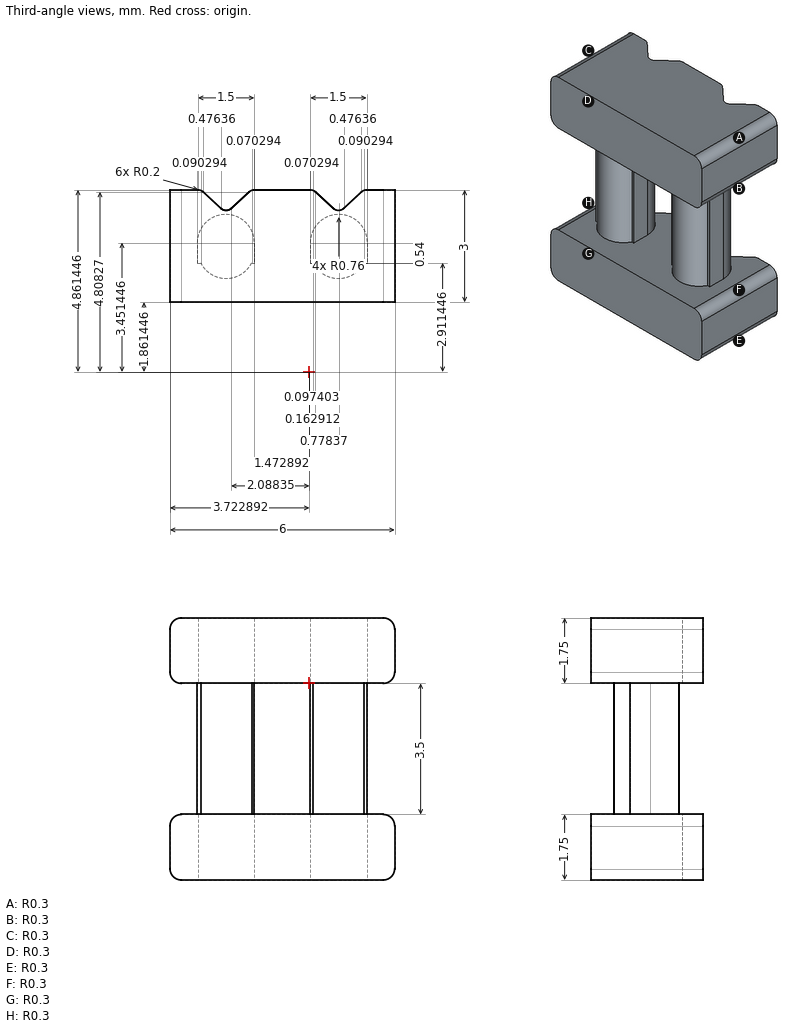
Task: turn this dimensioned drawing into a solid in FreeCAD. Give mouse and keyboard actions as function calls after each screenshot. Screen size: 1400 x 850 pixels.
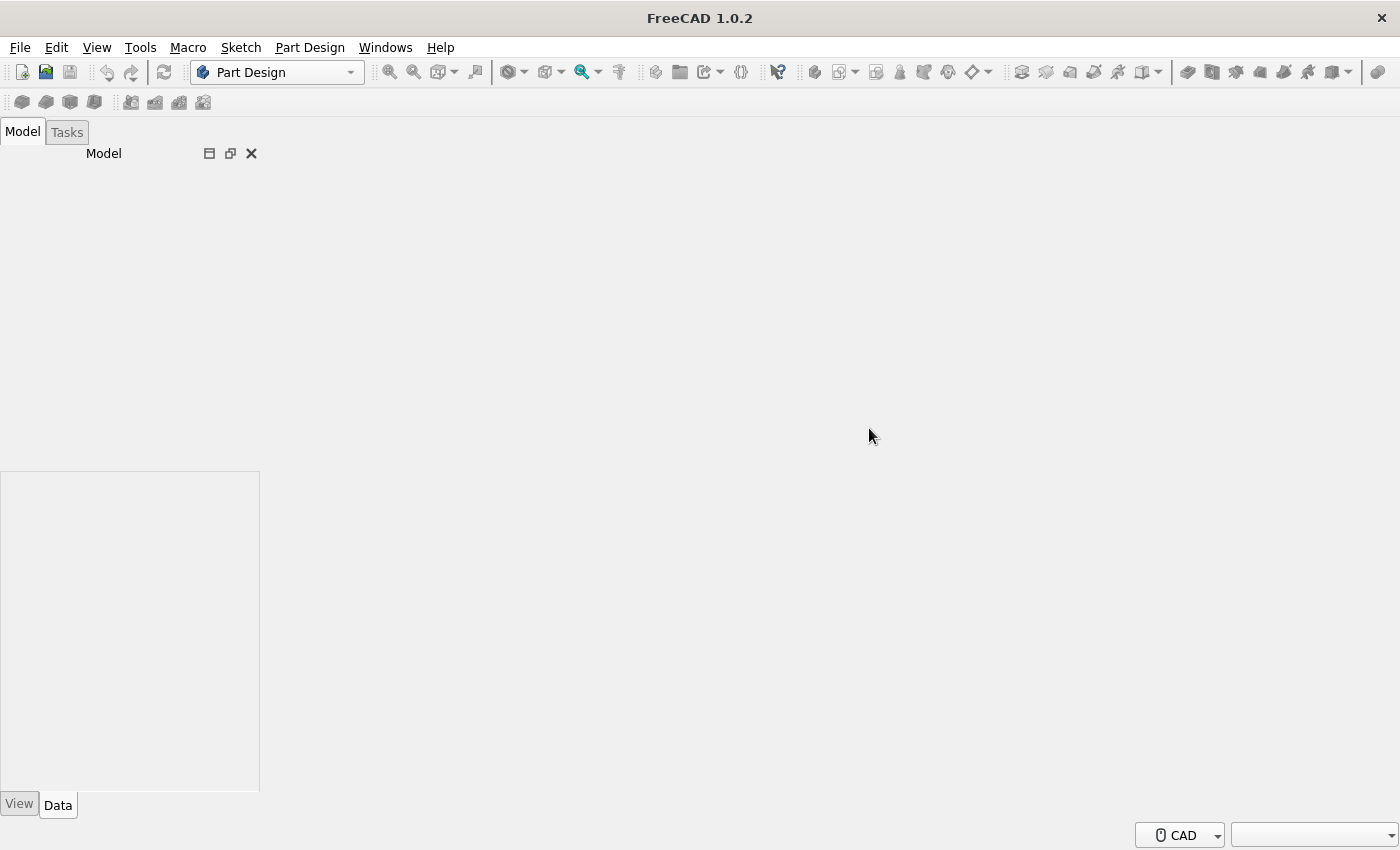
key(ctrl+n)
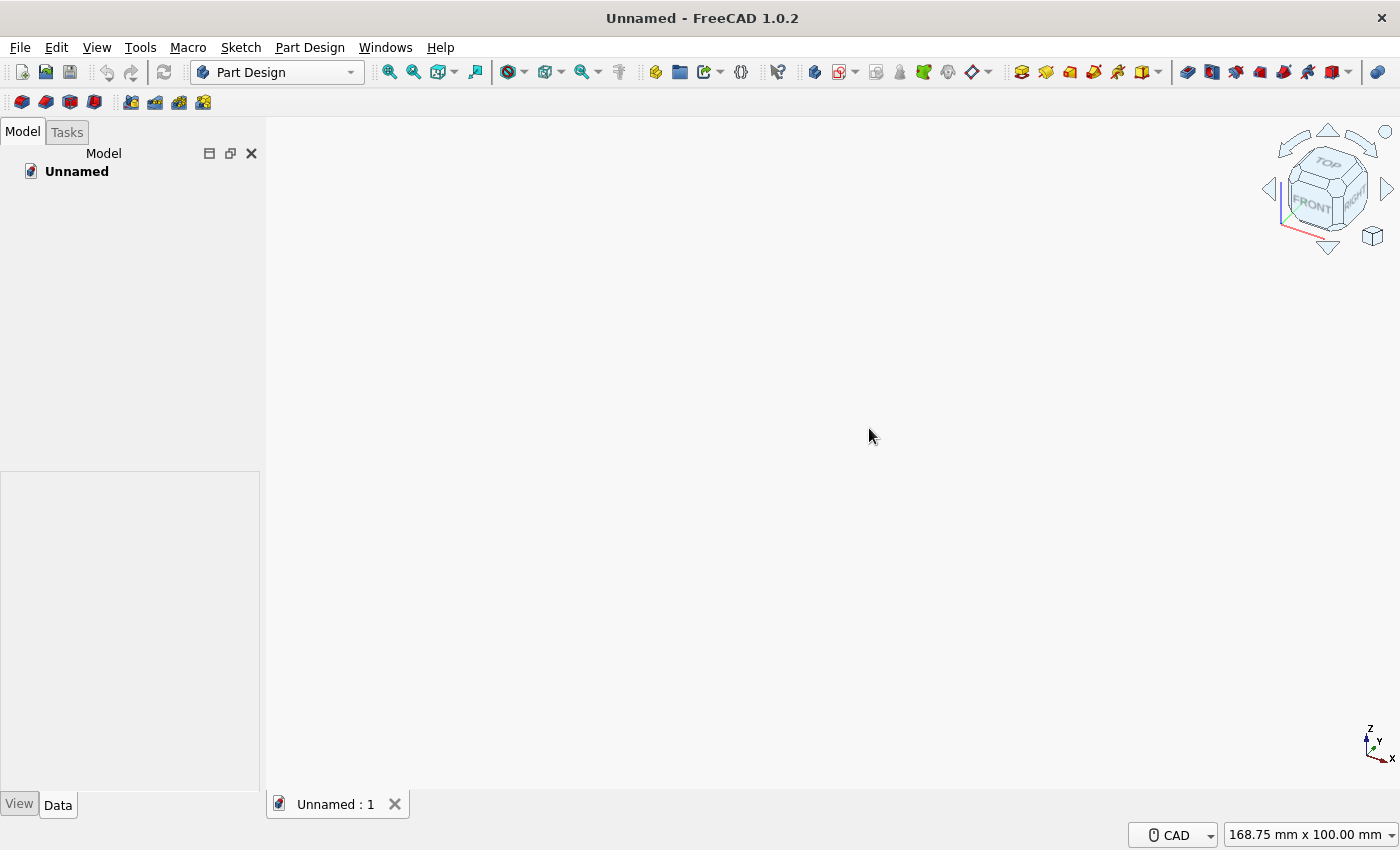
click(840, 72)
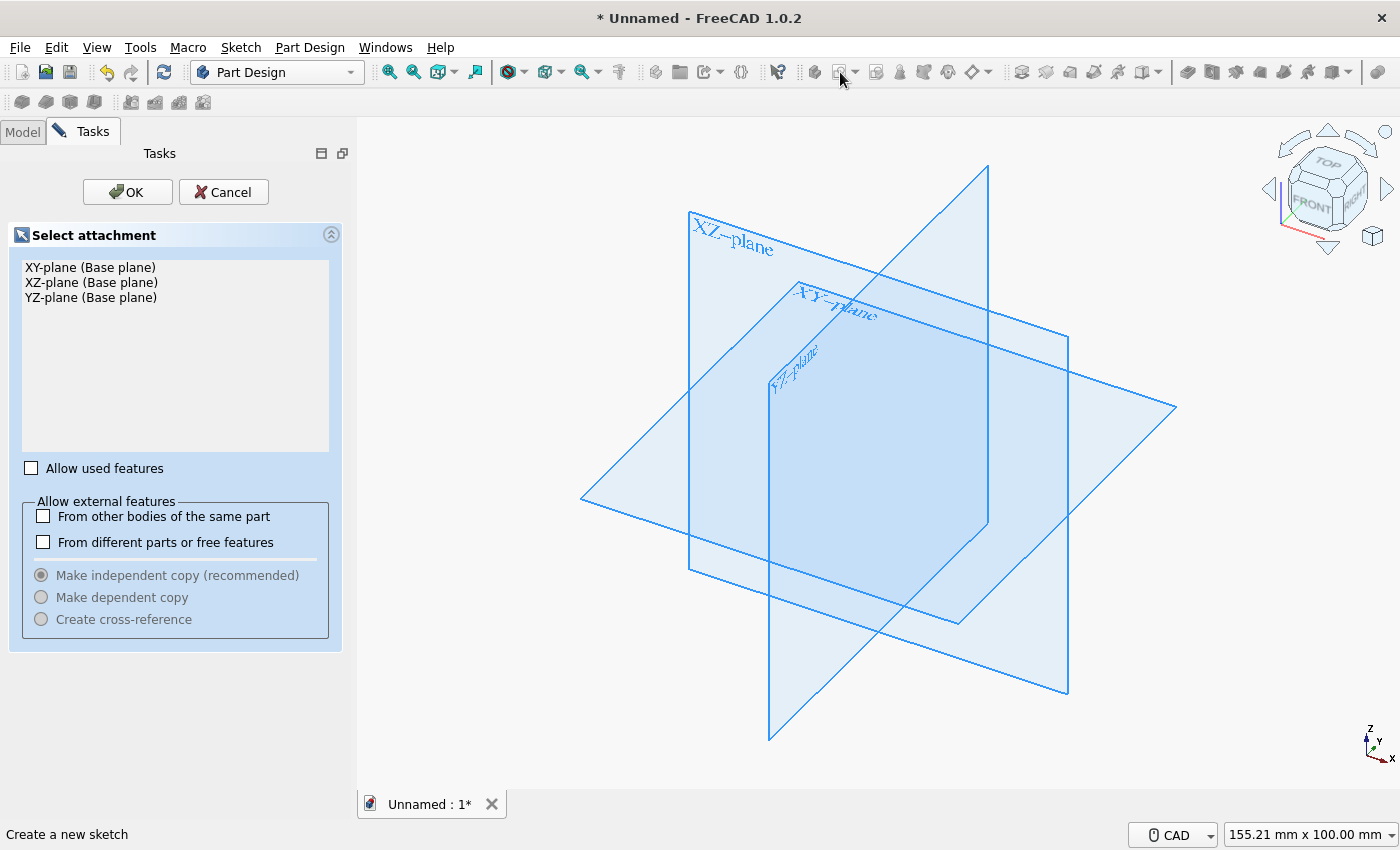
click(82, 268)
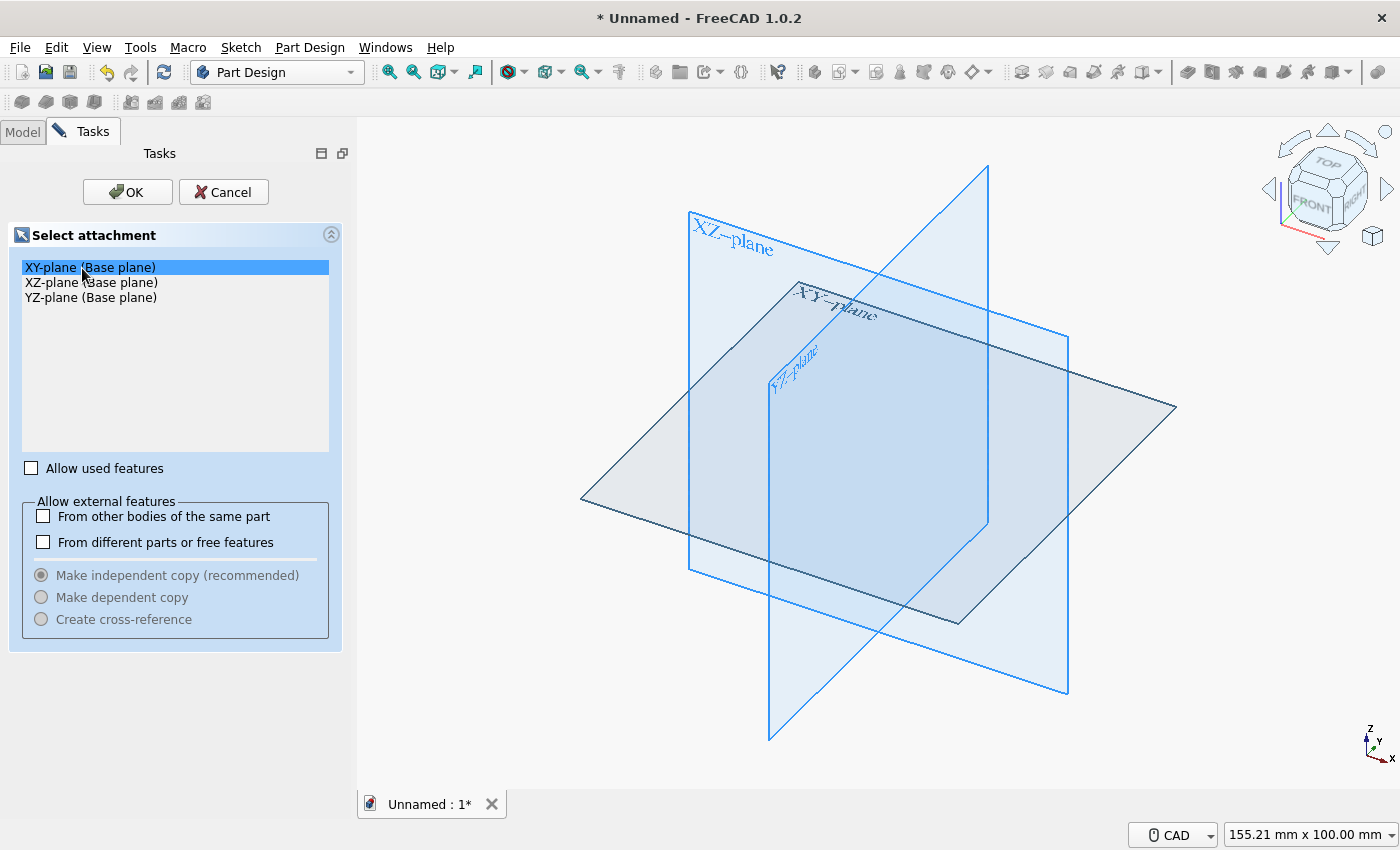
click(128, 192)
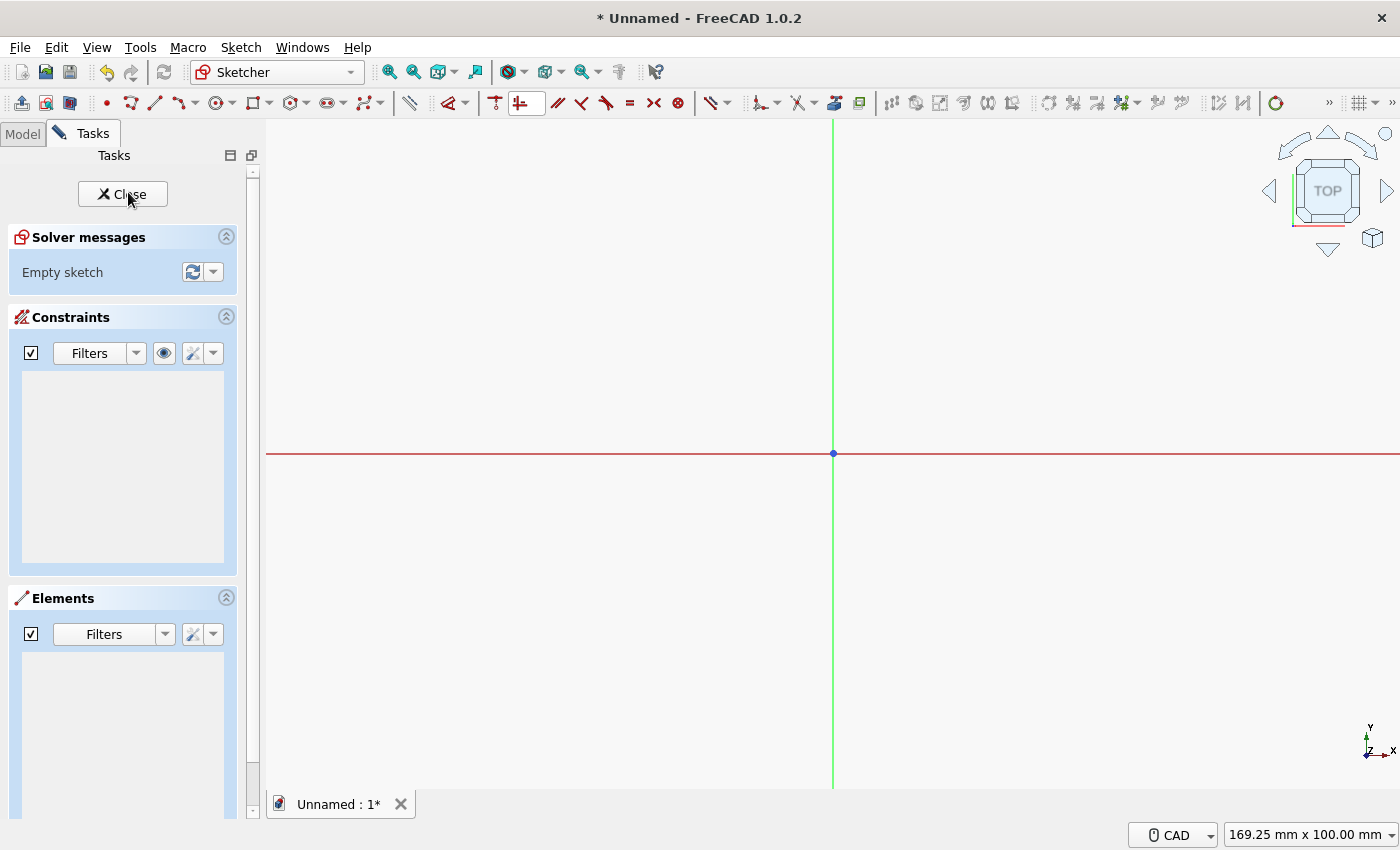
scroll(833, 436, up, 13)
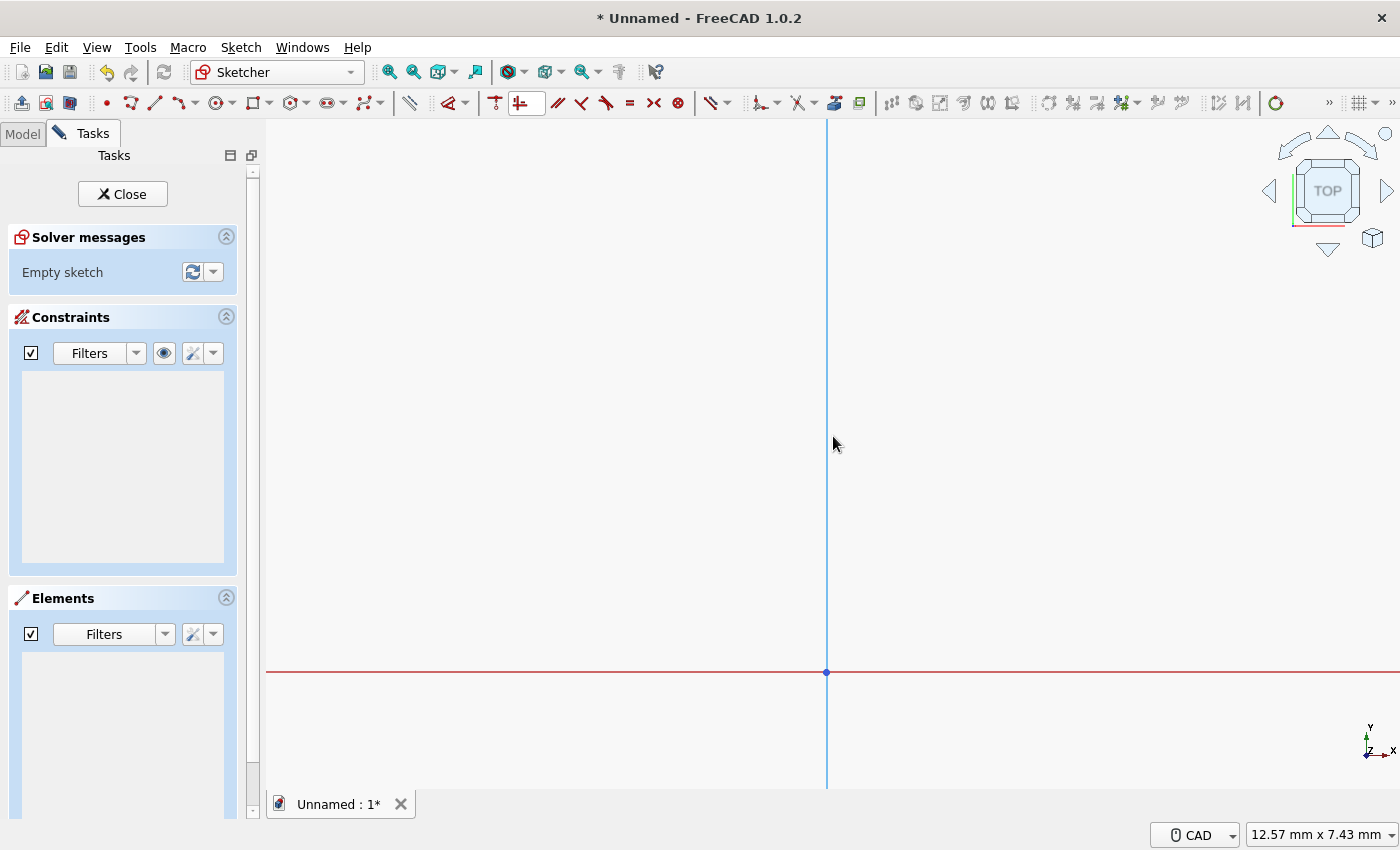
click(254, 104)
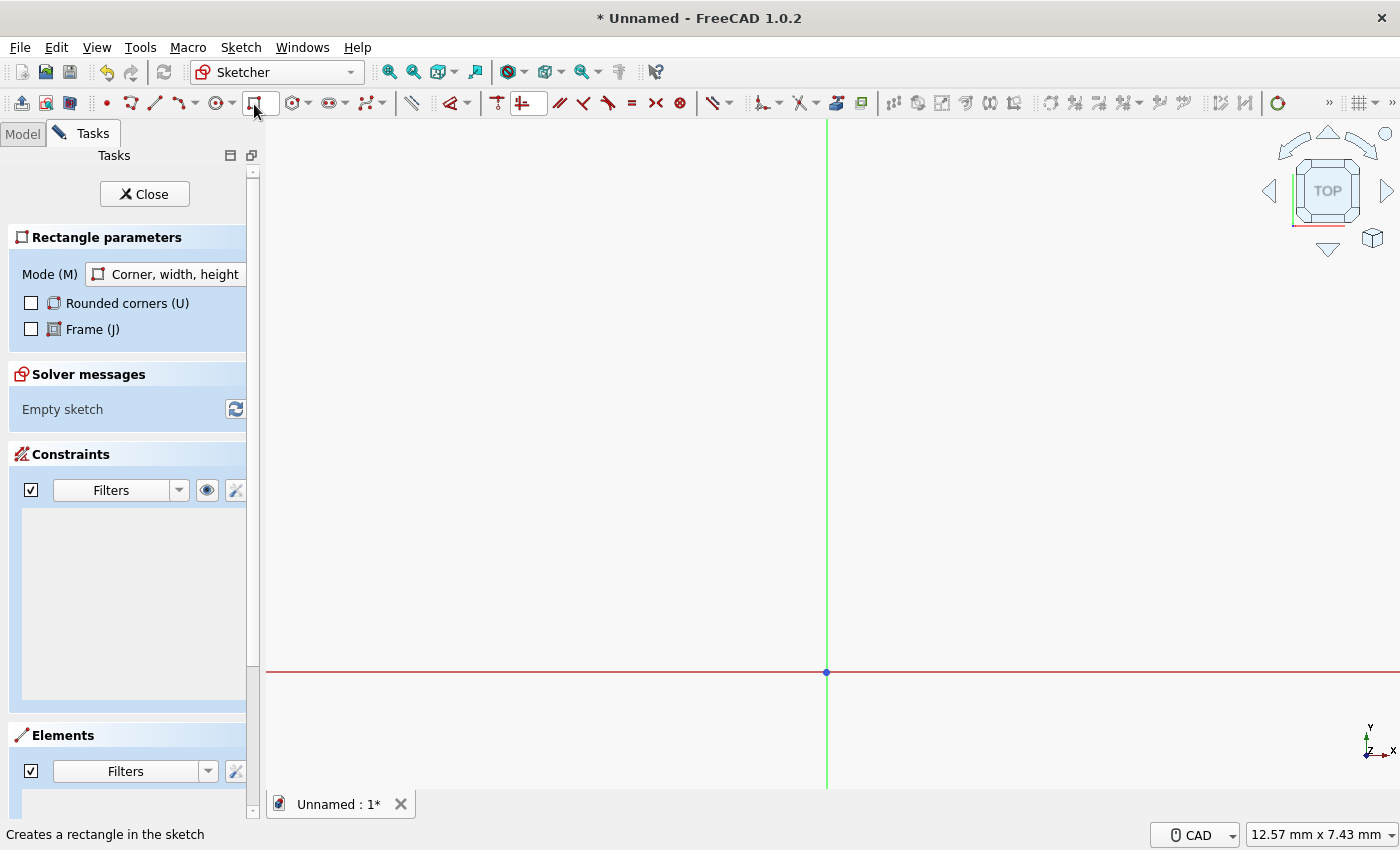
click(491, 234)
move(1032, 505)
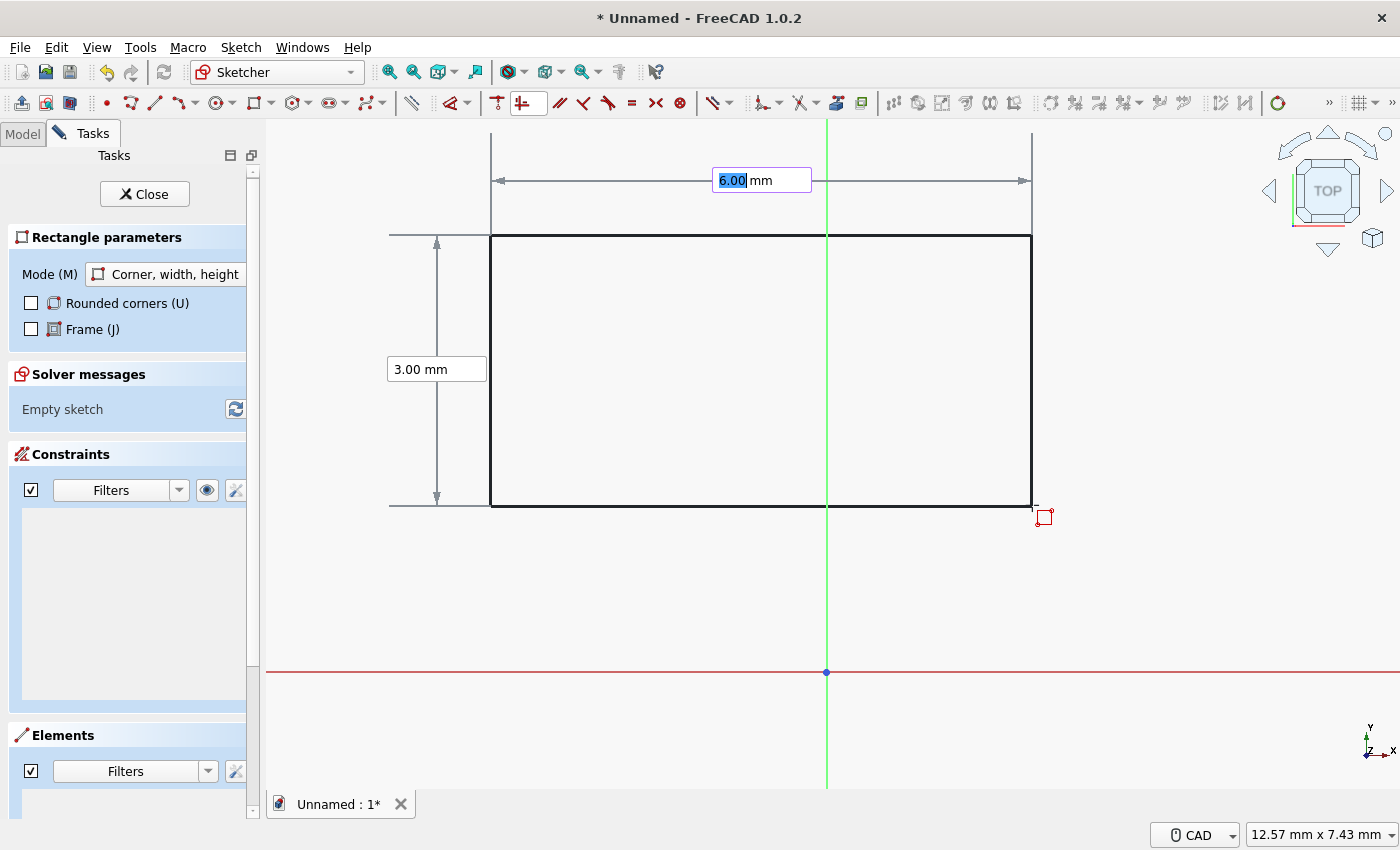
text(6)
key(Tab)
text(3)
key(Return)
key(Escape)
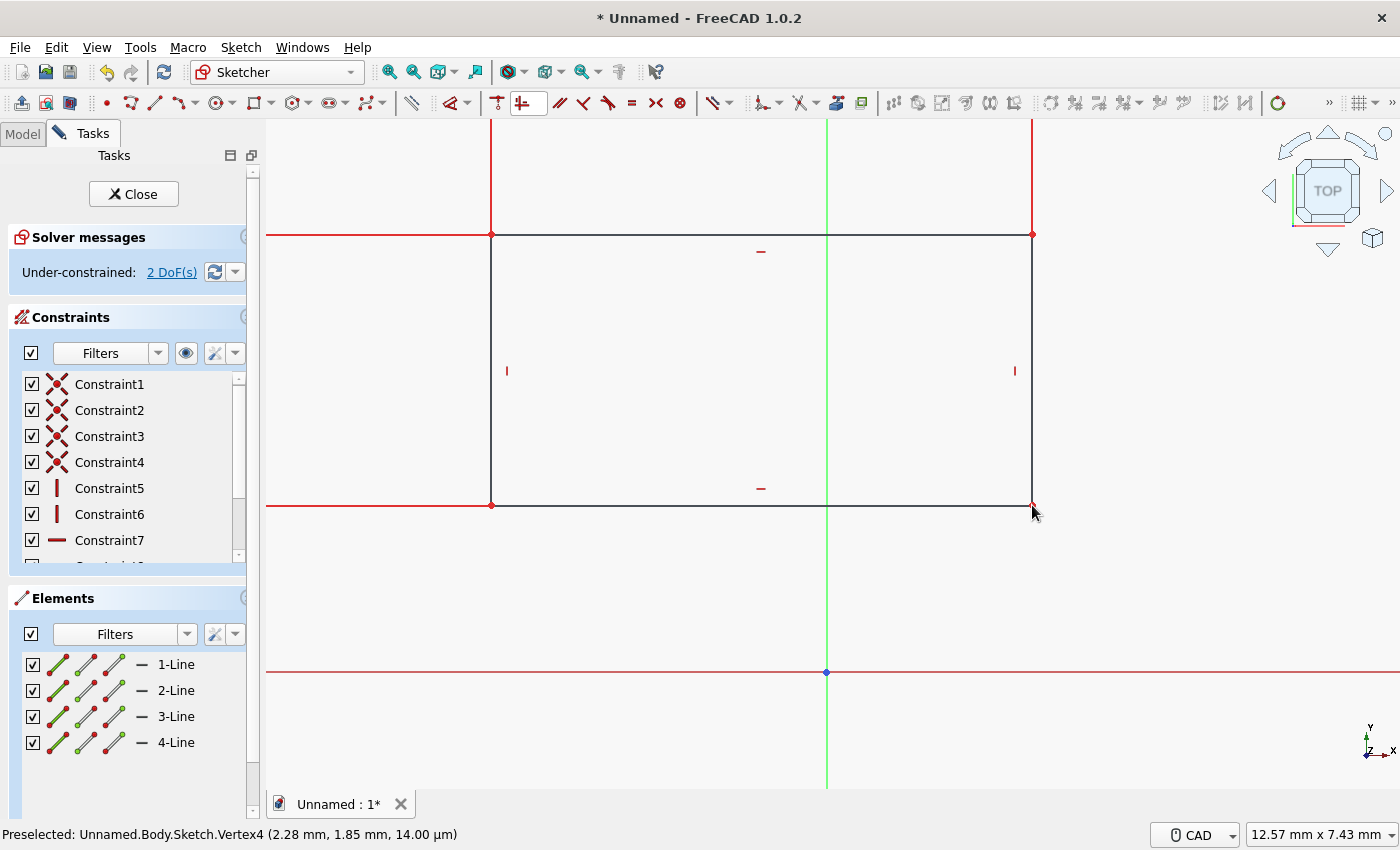
click(491, 235)